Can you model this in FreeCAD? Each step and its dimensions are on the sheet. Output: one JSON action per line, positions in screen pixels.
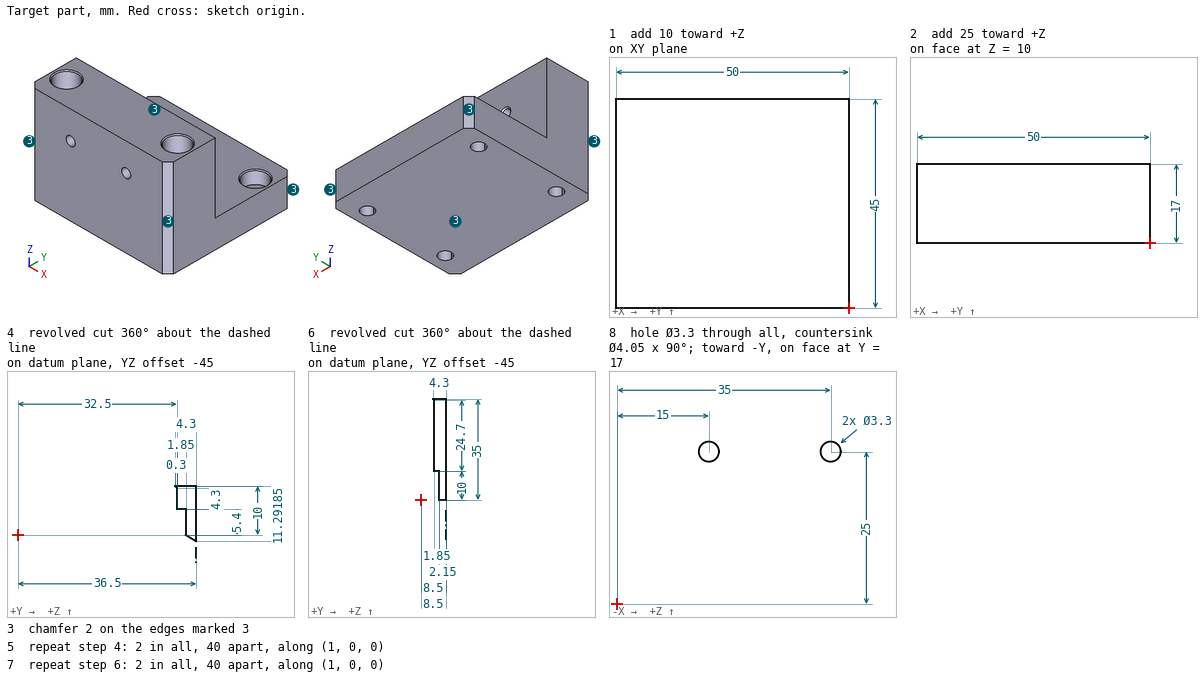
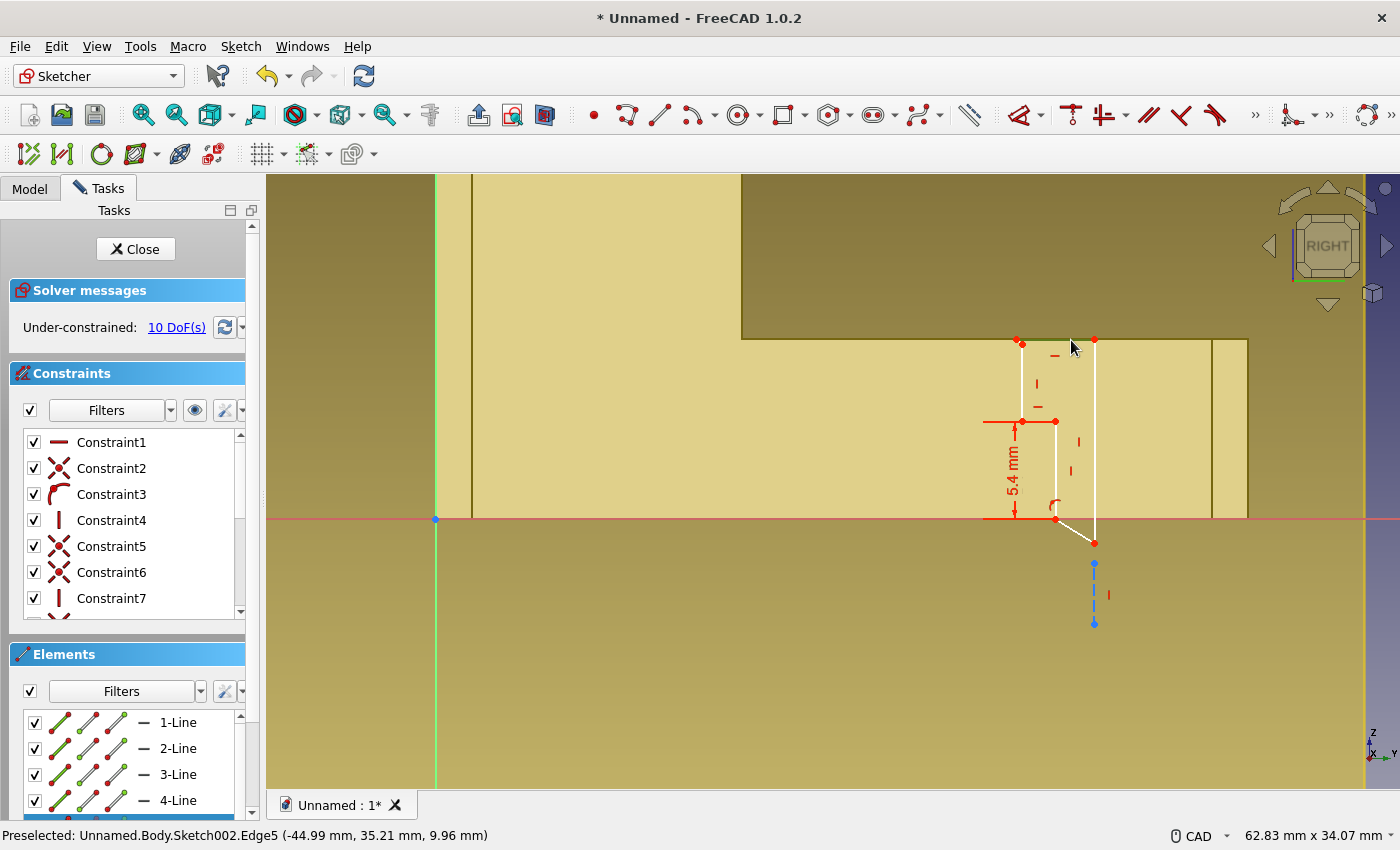
{"action": "key", "text": "l"}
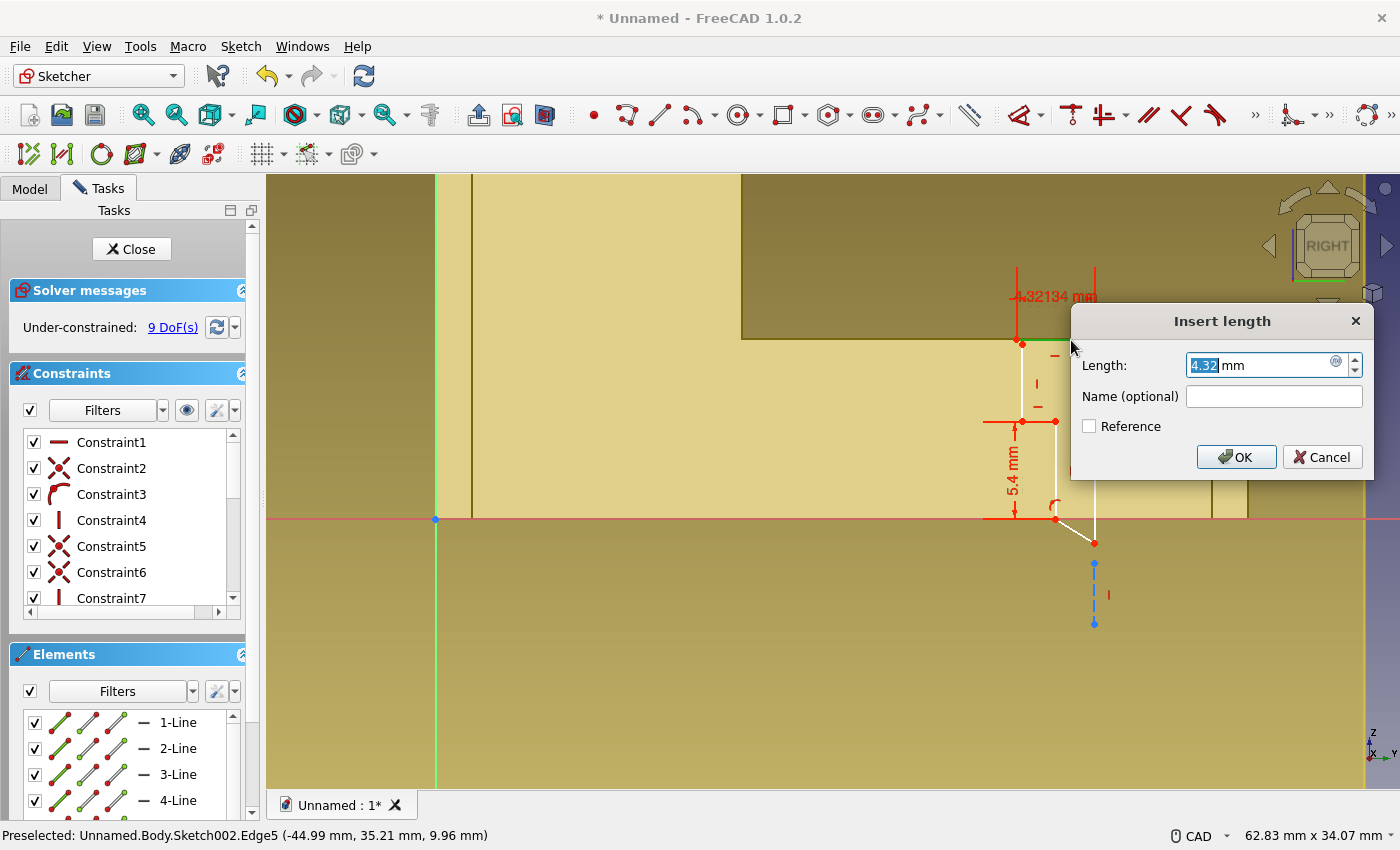
{"action": "type", "text": "4.3"}
{"action": "key", "text": "Return"}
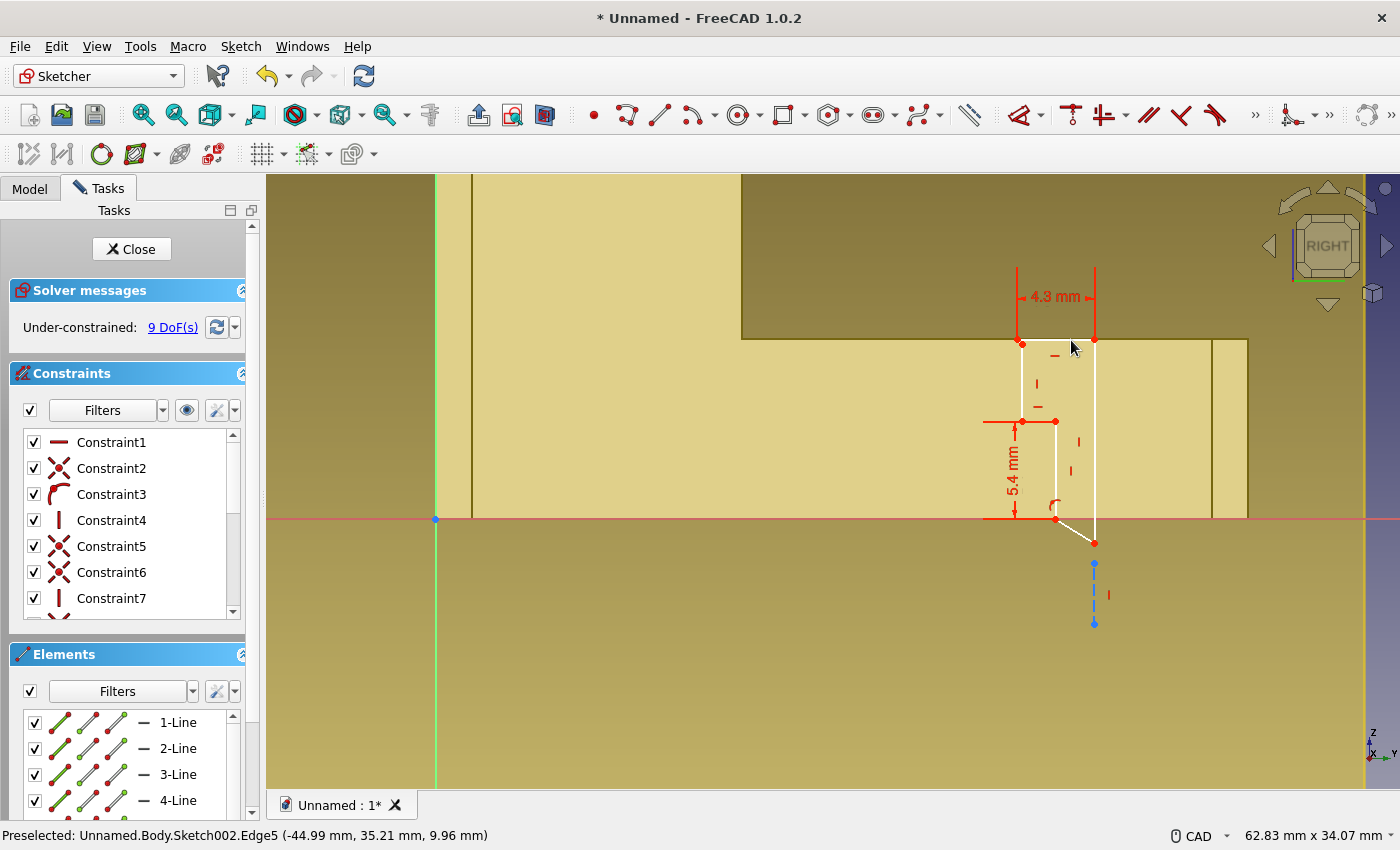
{"action": "left_click", "coordinate": [1022, 368]}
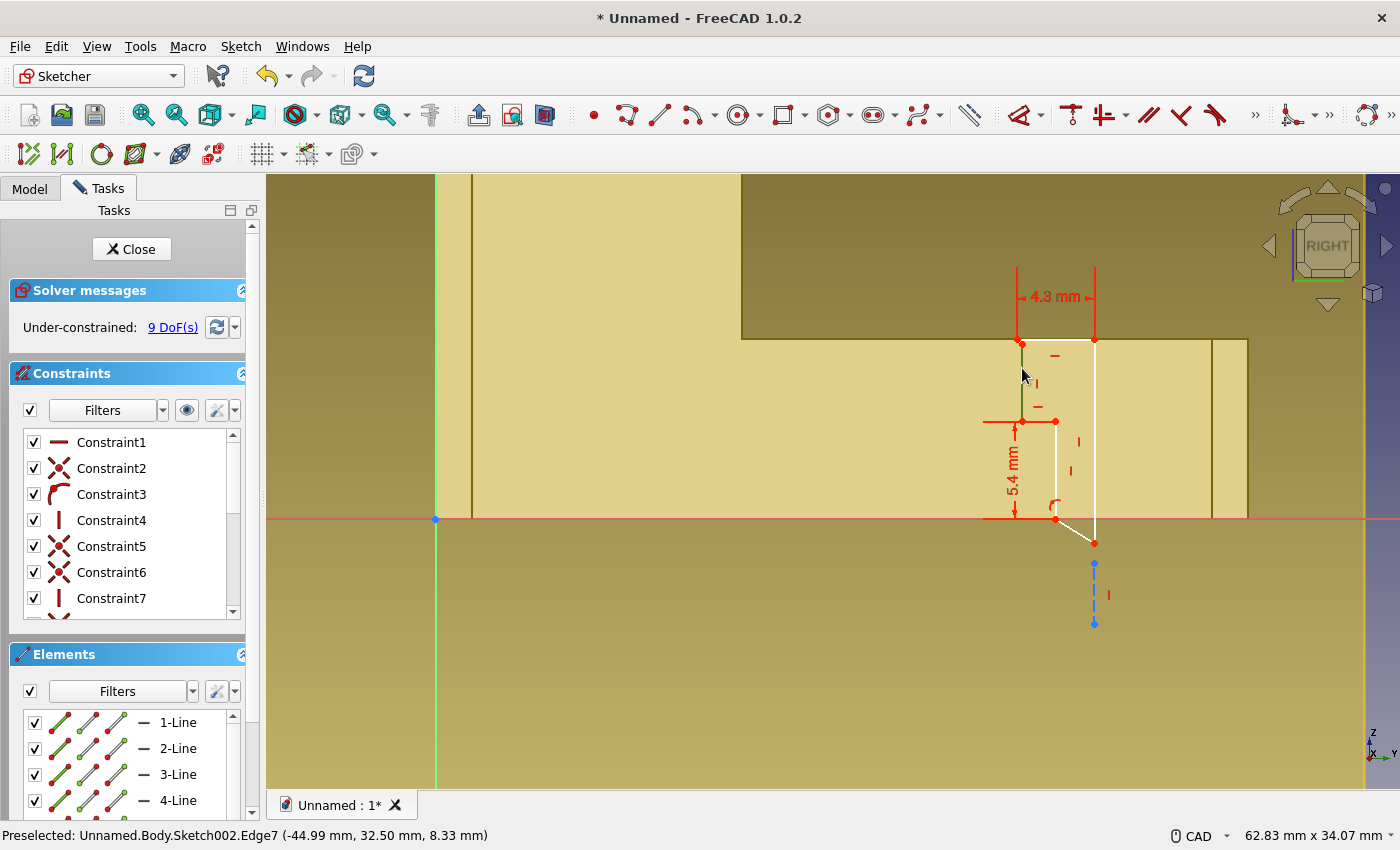
{"action": "key", "text": "i"}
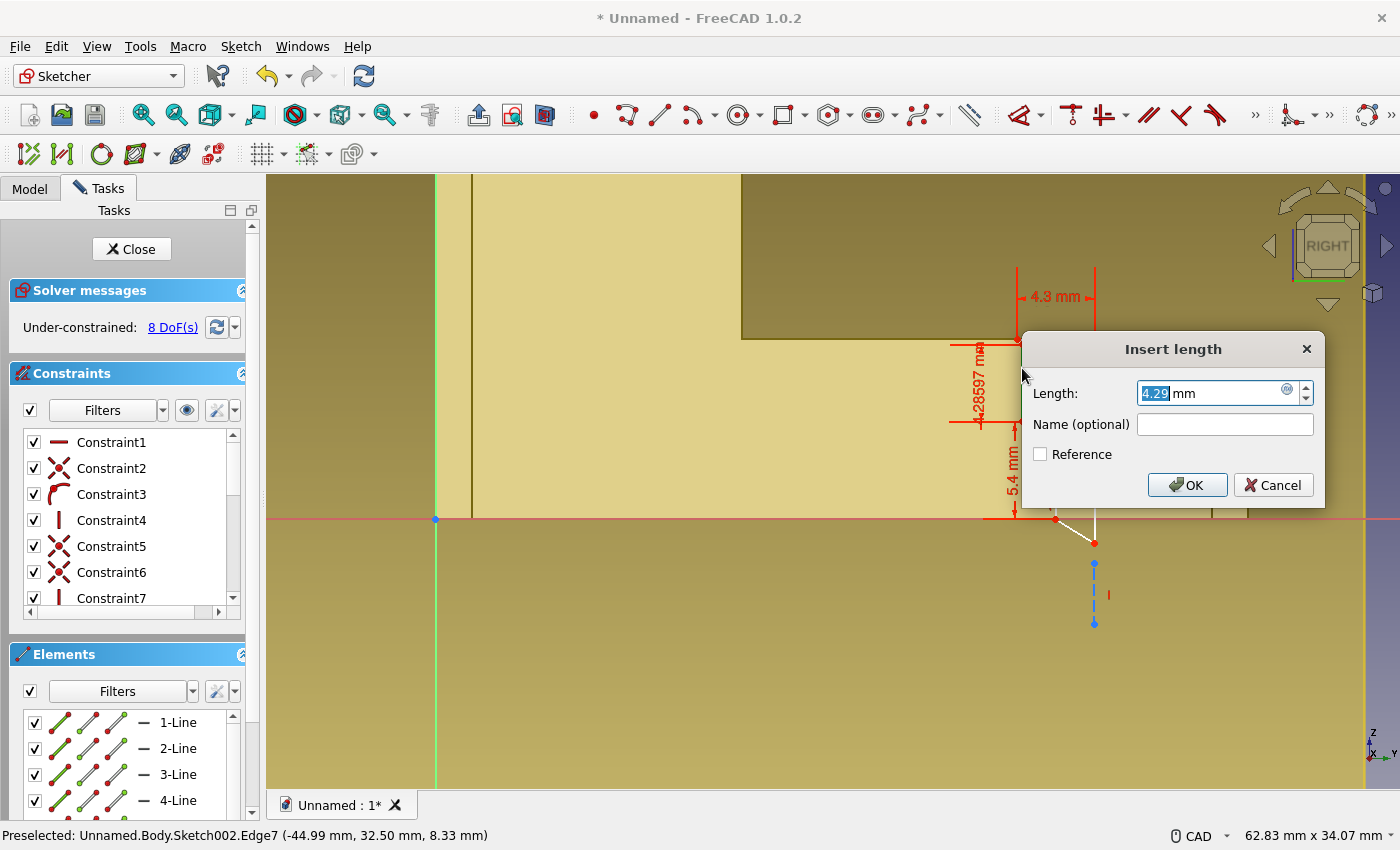
{"action": "type", "text": "4.3"}
{"action": "key", "text": "Return"}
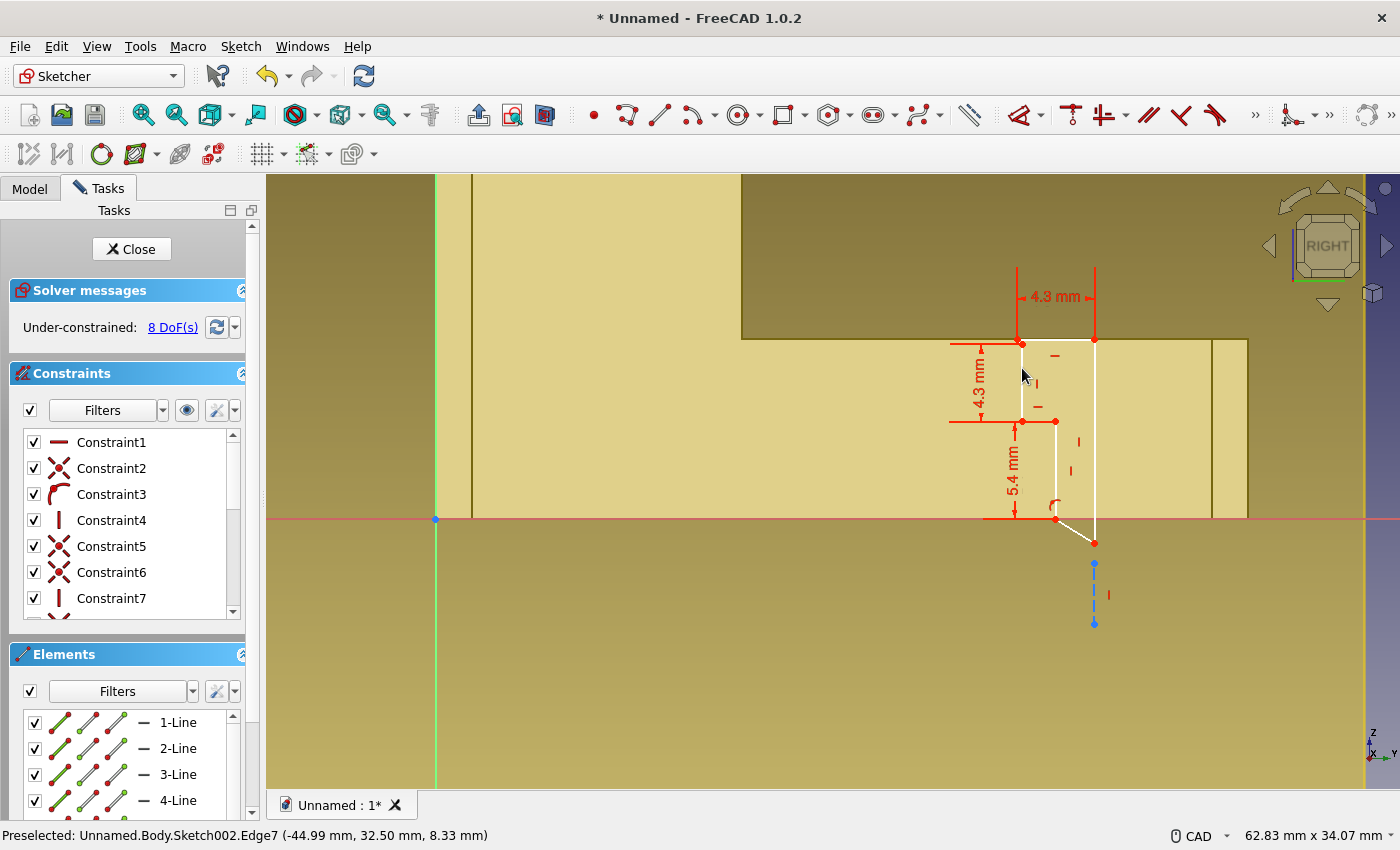
{"action": "left_click", "coordinate": [1095, 340]}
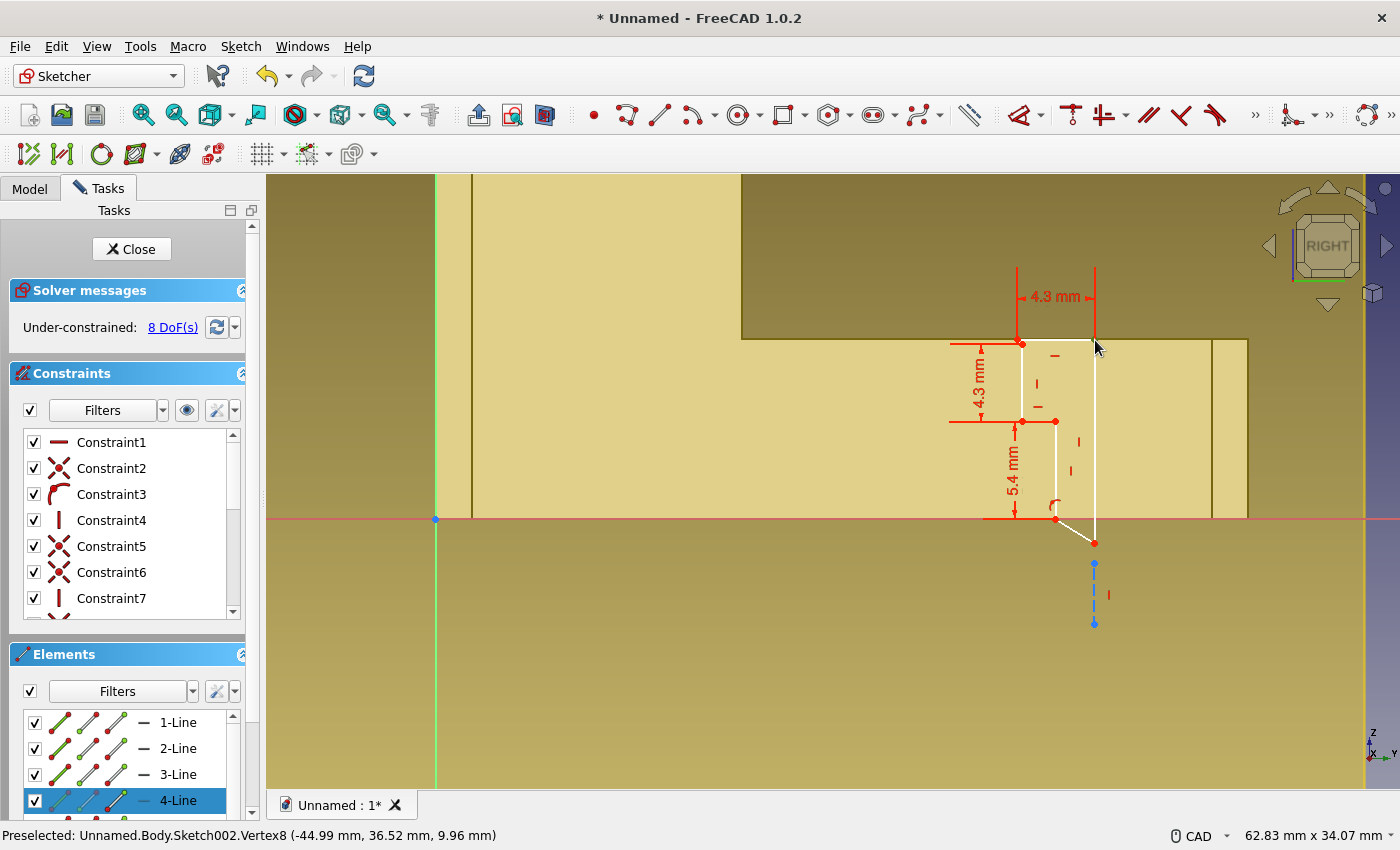
{"action": "key", "text": "i"}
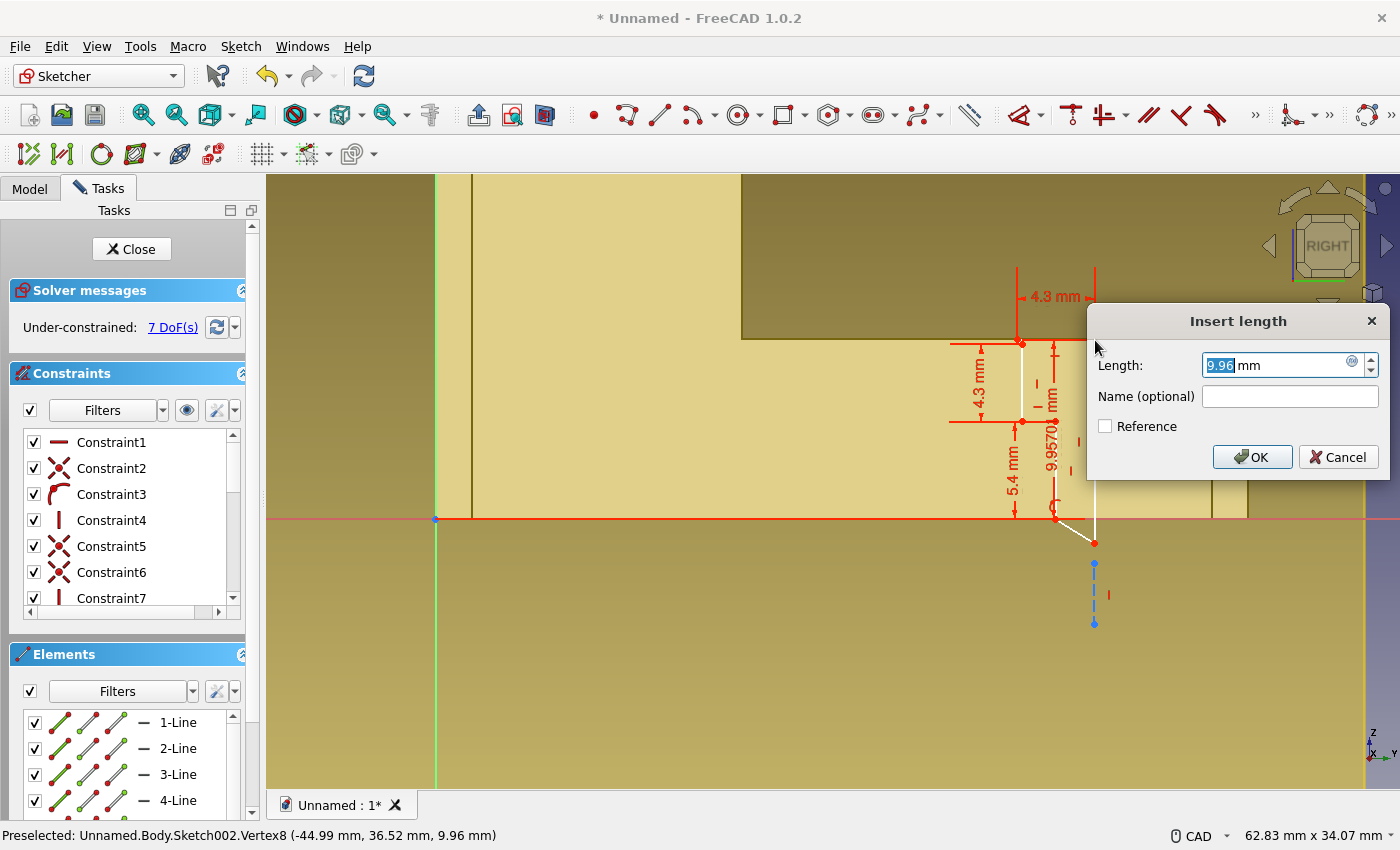
{"action": "type", "text": "10"}
{"action": "key", "text": "Return"}